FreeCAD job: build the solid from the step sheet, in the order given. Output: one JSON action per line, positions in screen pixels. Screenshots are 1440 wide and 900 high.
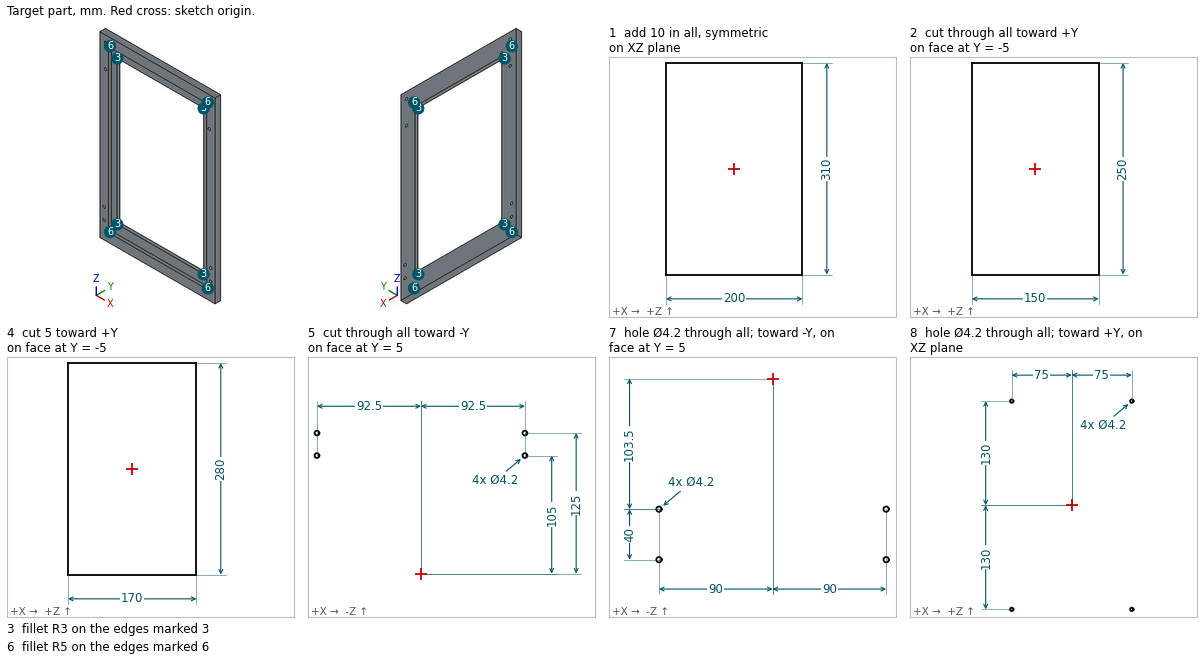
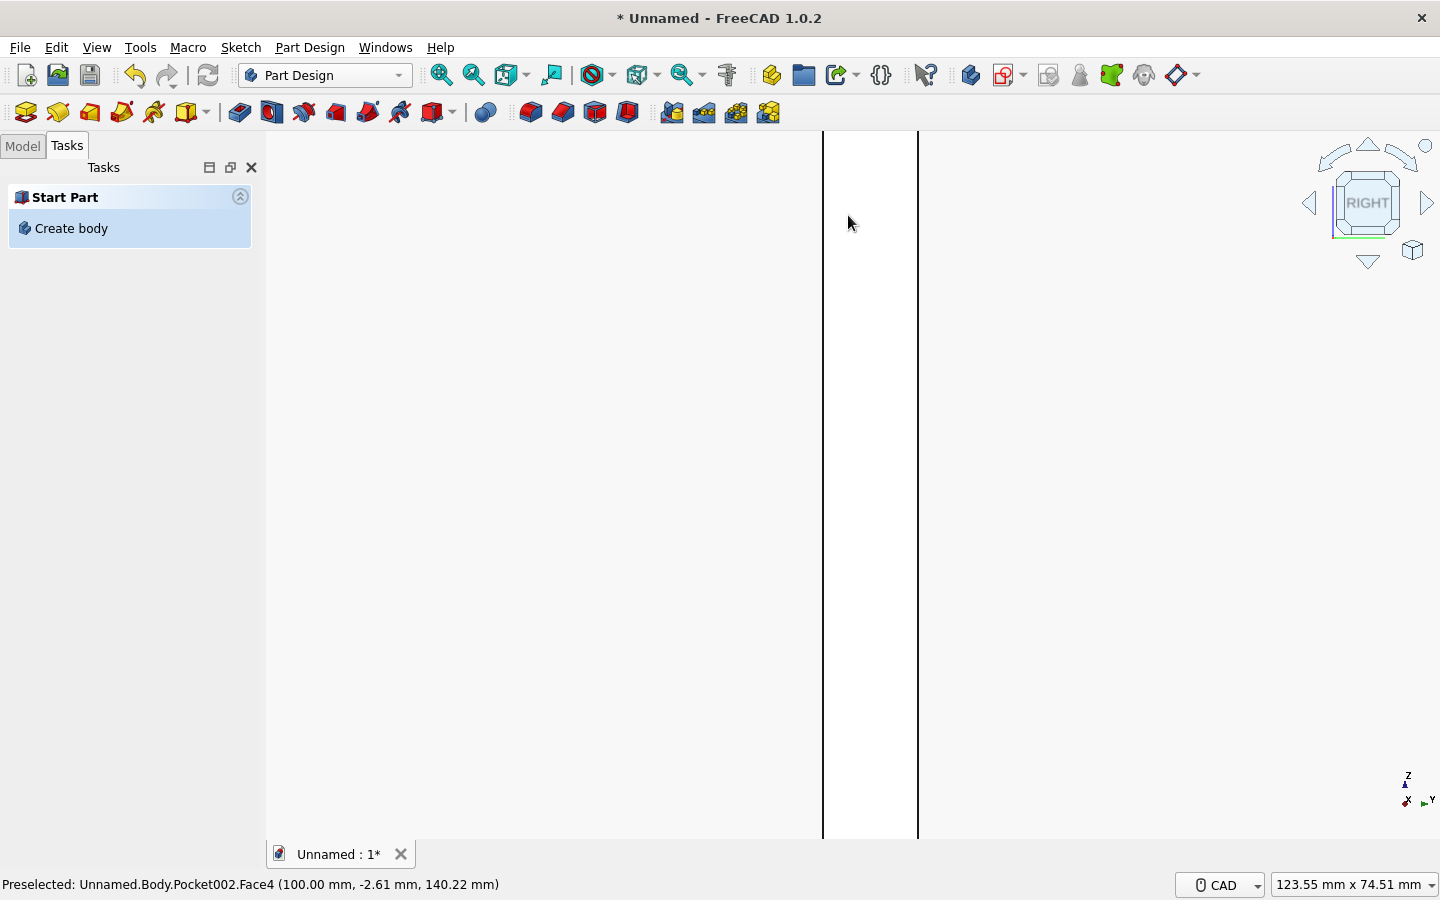
{"action": "left_click", "coordinate": [442, 76]}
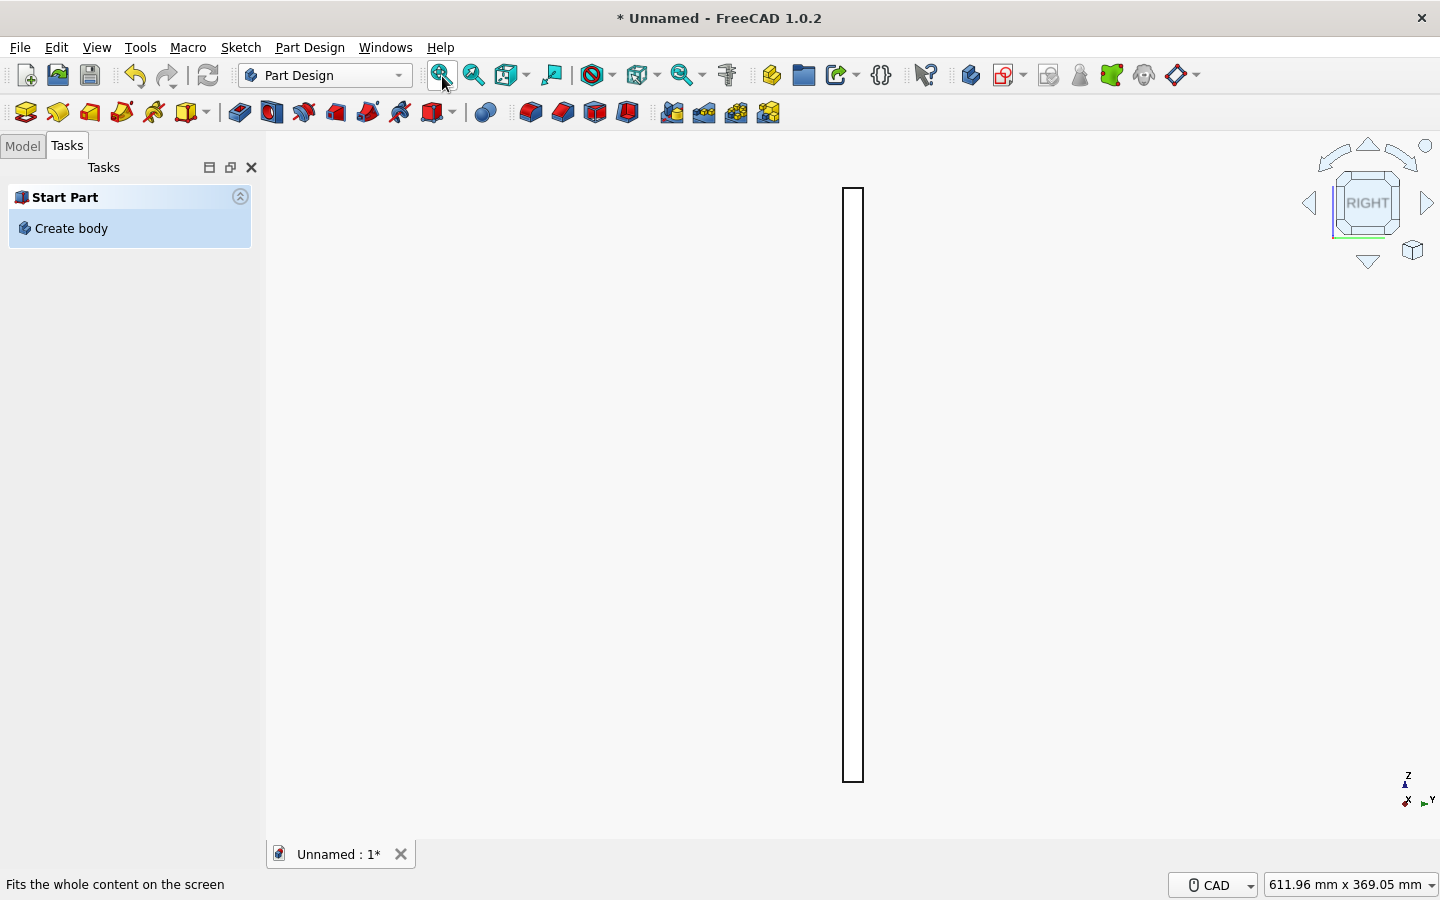
{"action": "key", "text": "5"}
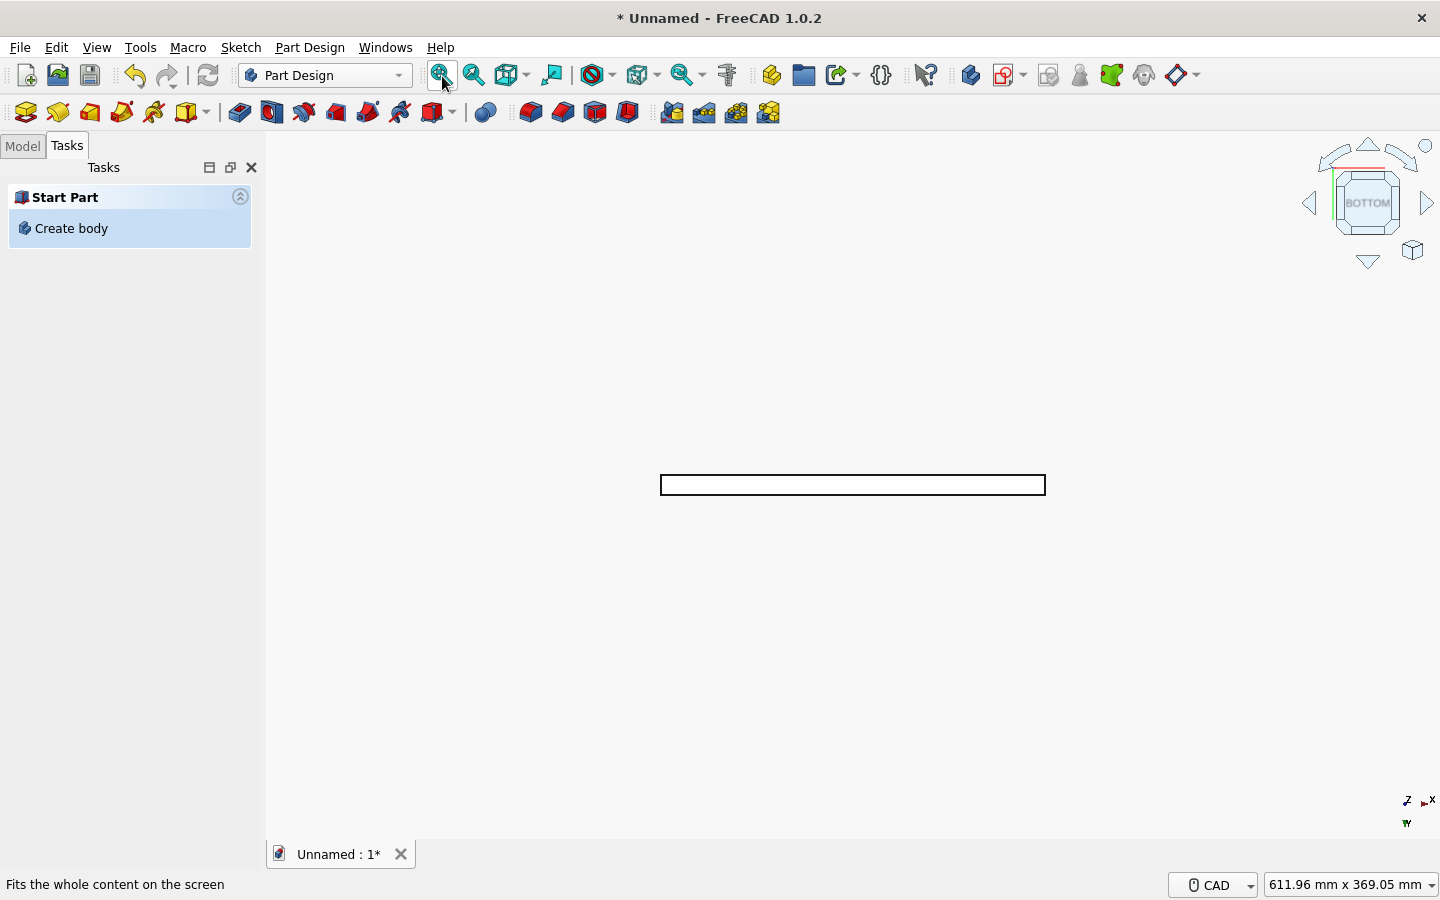
{"action": "key", "text": "v f"}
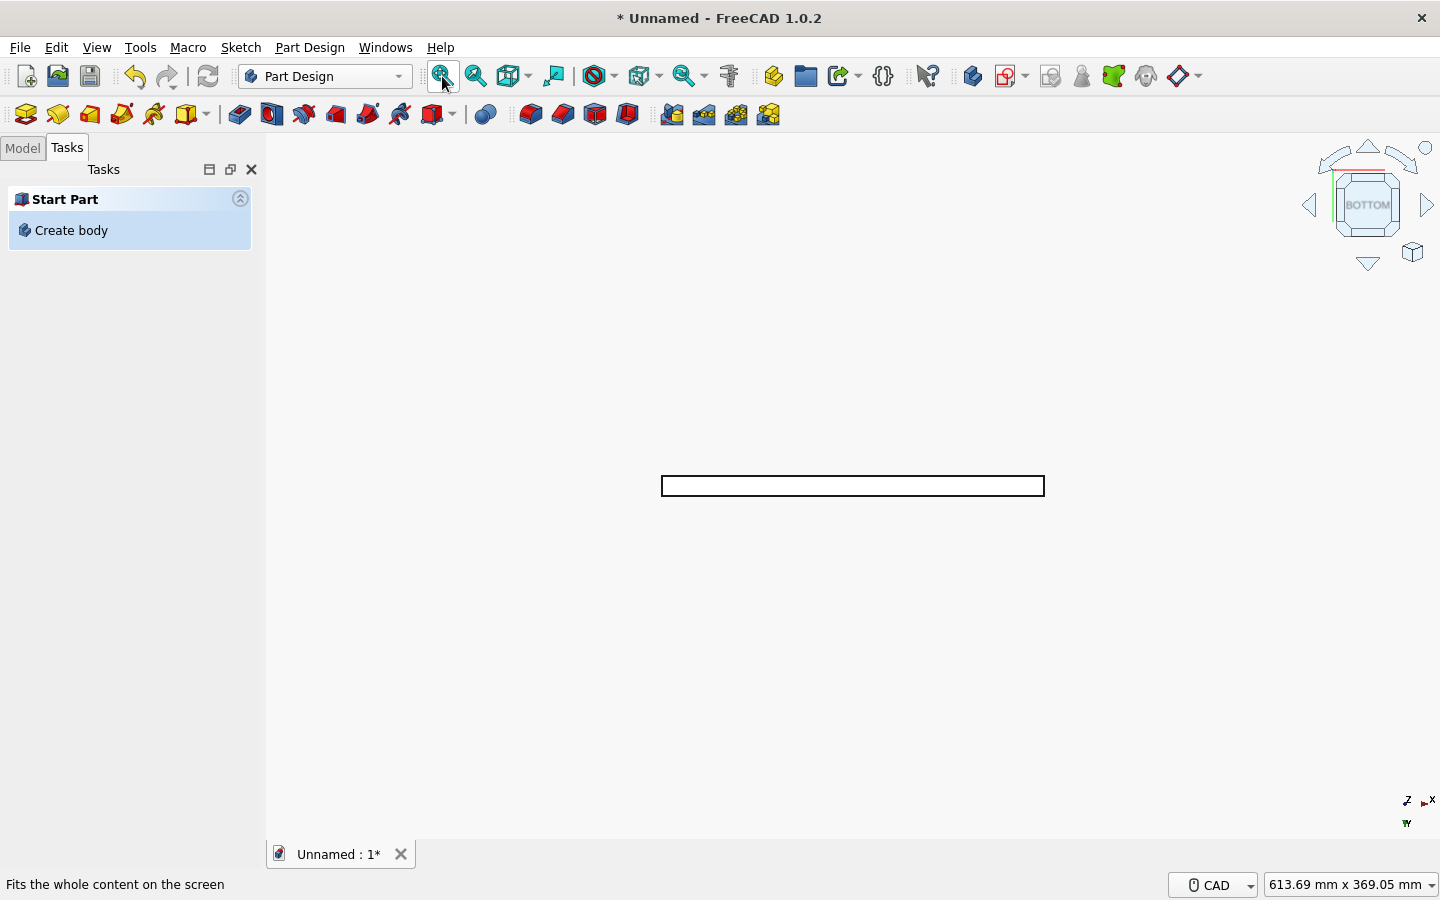
{"action": "scroll", "coordinate": [1016, 480], "scroll_direction": "up", "scroll_amount": 8}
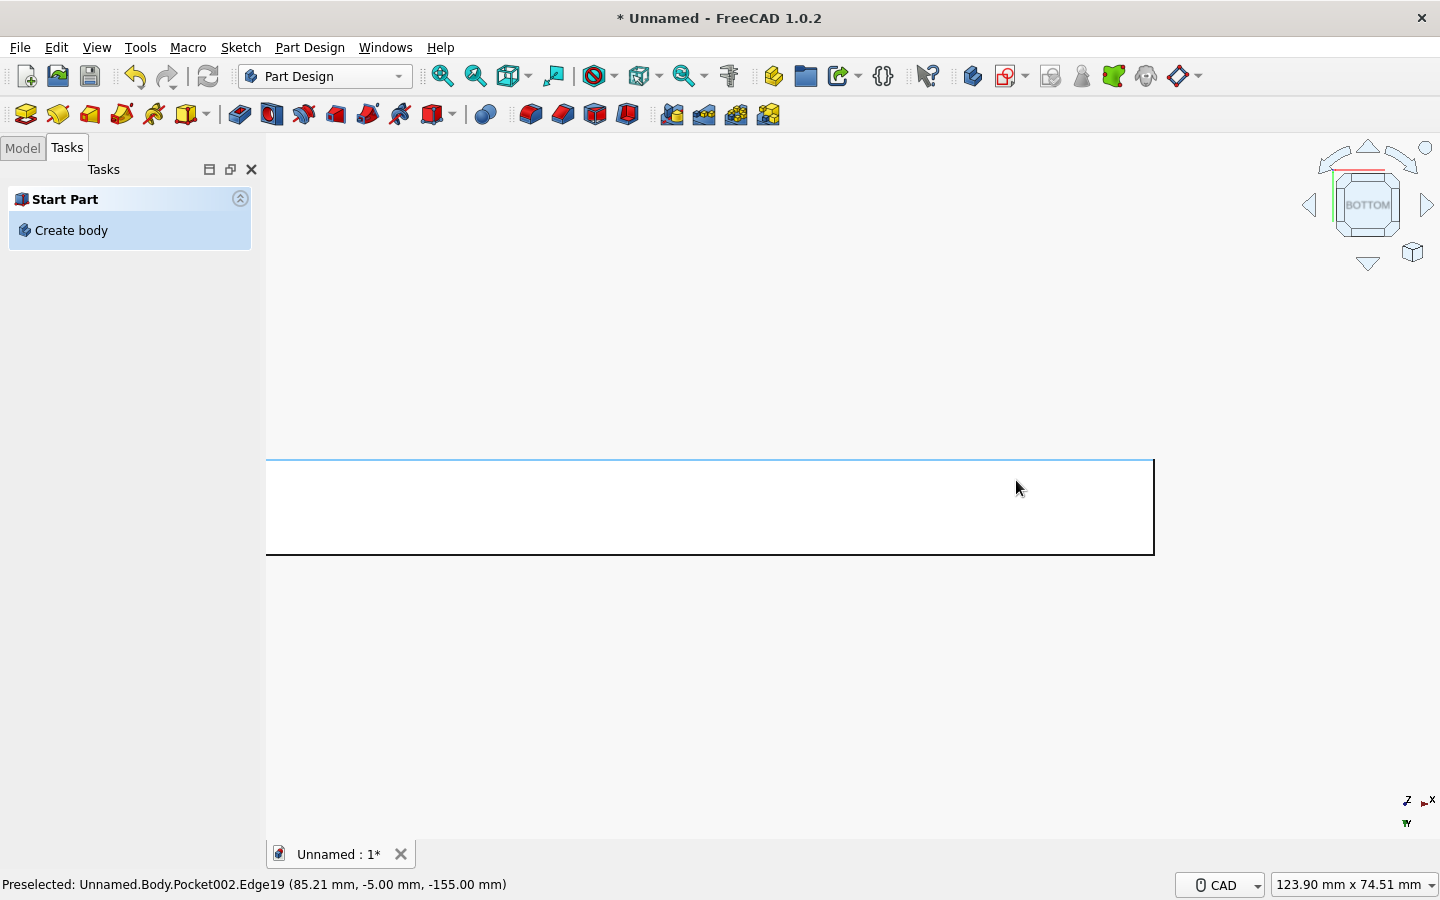
{"action": "left_click", "coordinate": [444, 76]}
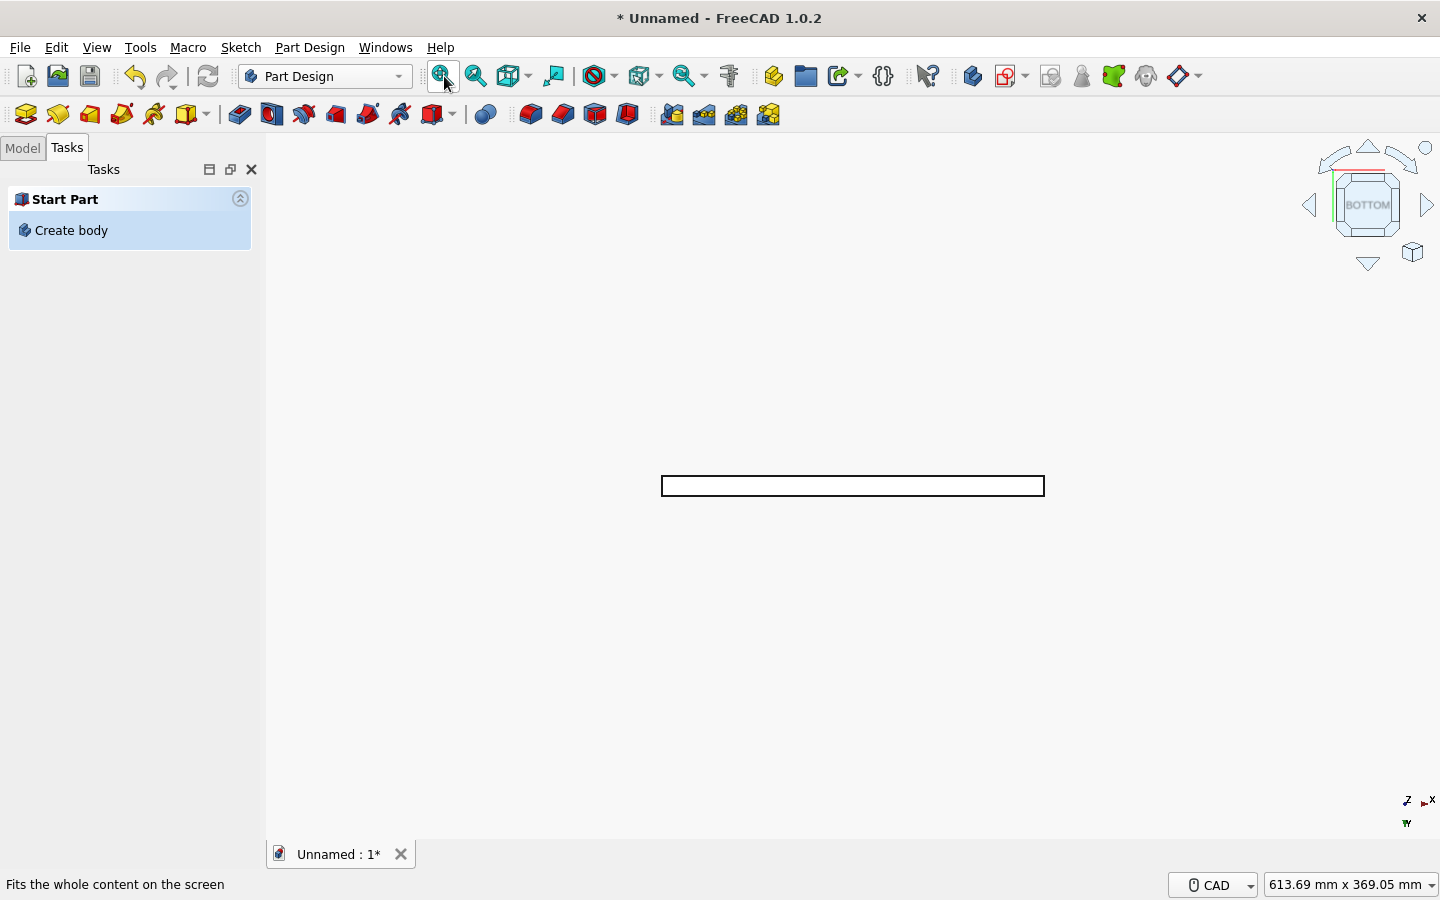
{"action": "key", "text": "4"}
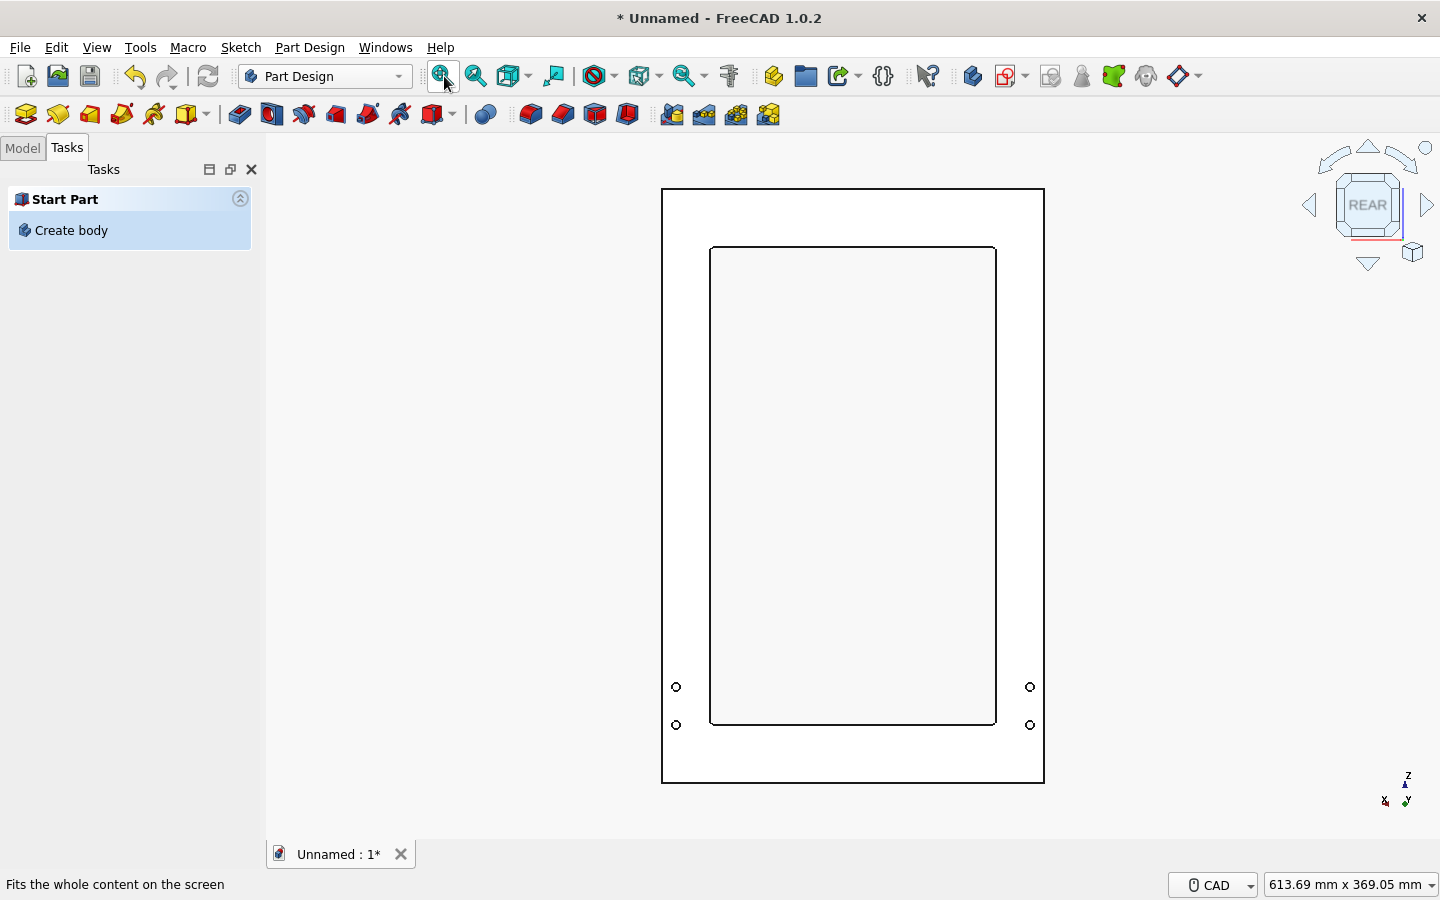
{"action": "scroll", "coordinate": [690, 217], "scroll_direction": "up", "scroll_amount": 8}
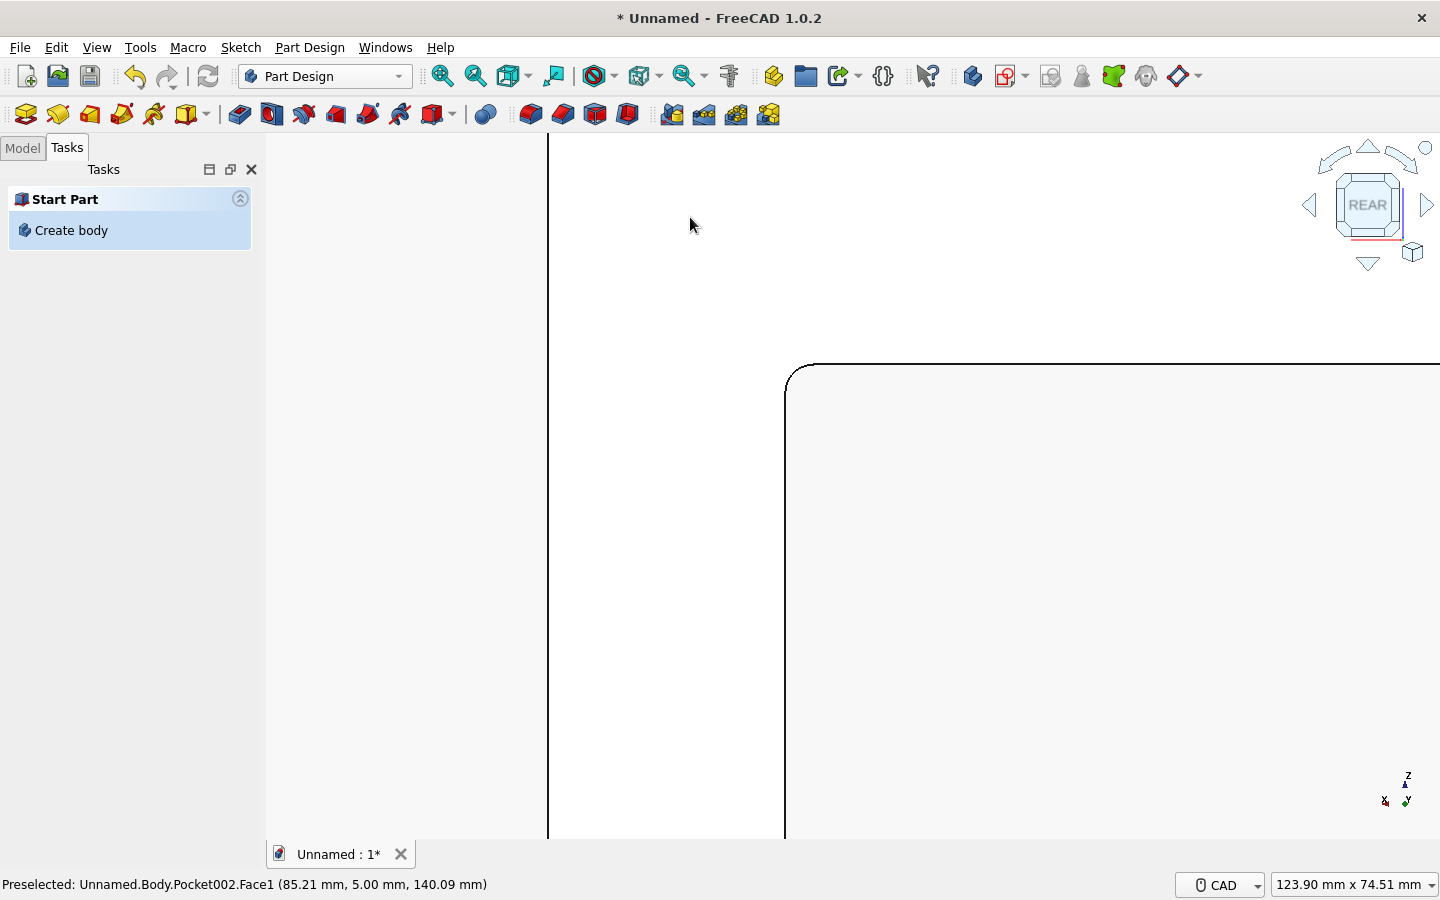
{"action": "left_click", "coordinate": [444, 76]}